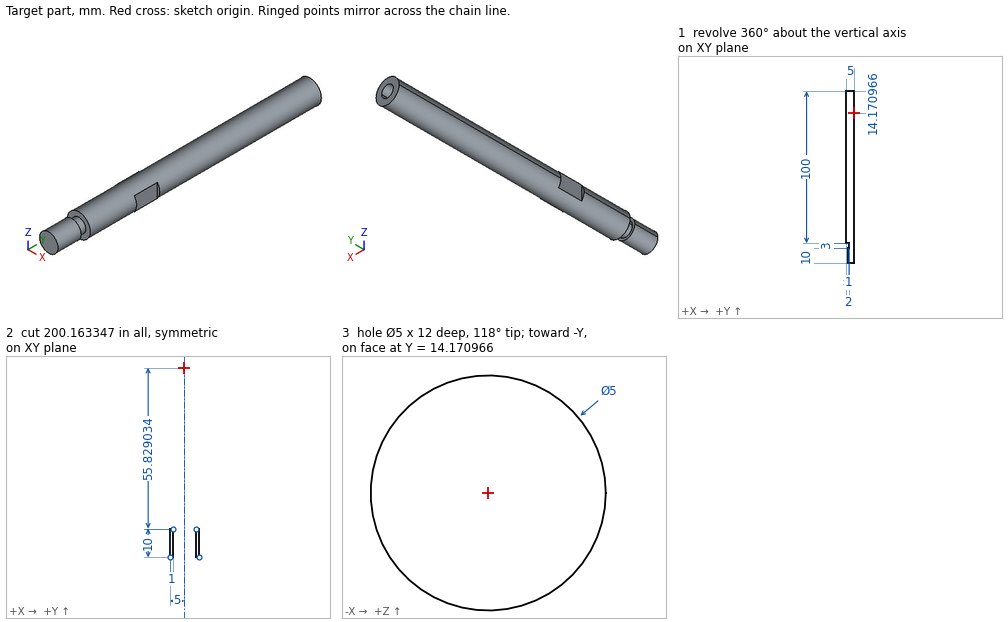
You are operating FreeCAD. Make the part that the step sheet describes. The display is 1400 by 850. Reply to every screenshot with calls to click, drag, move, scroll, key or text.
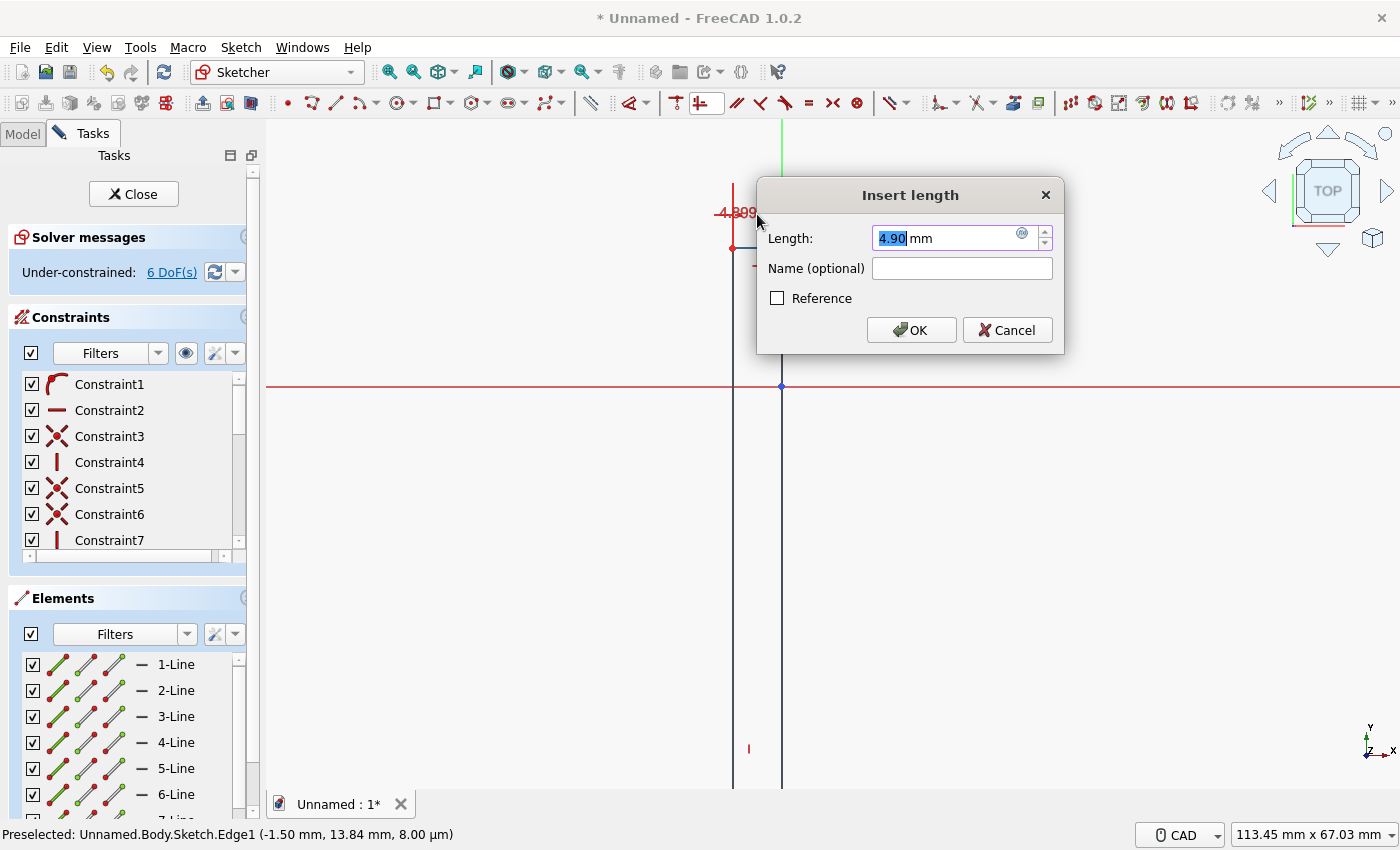
text(5)
key(Return)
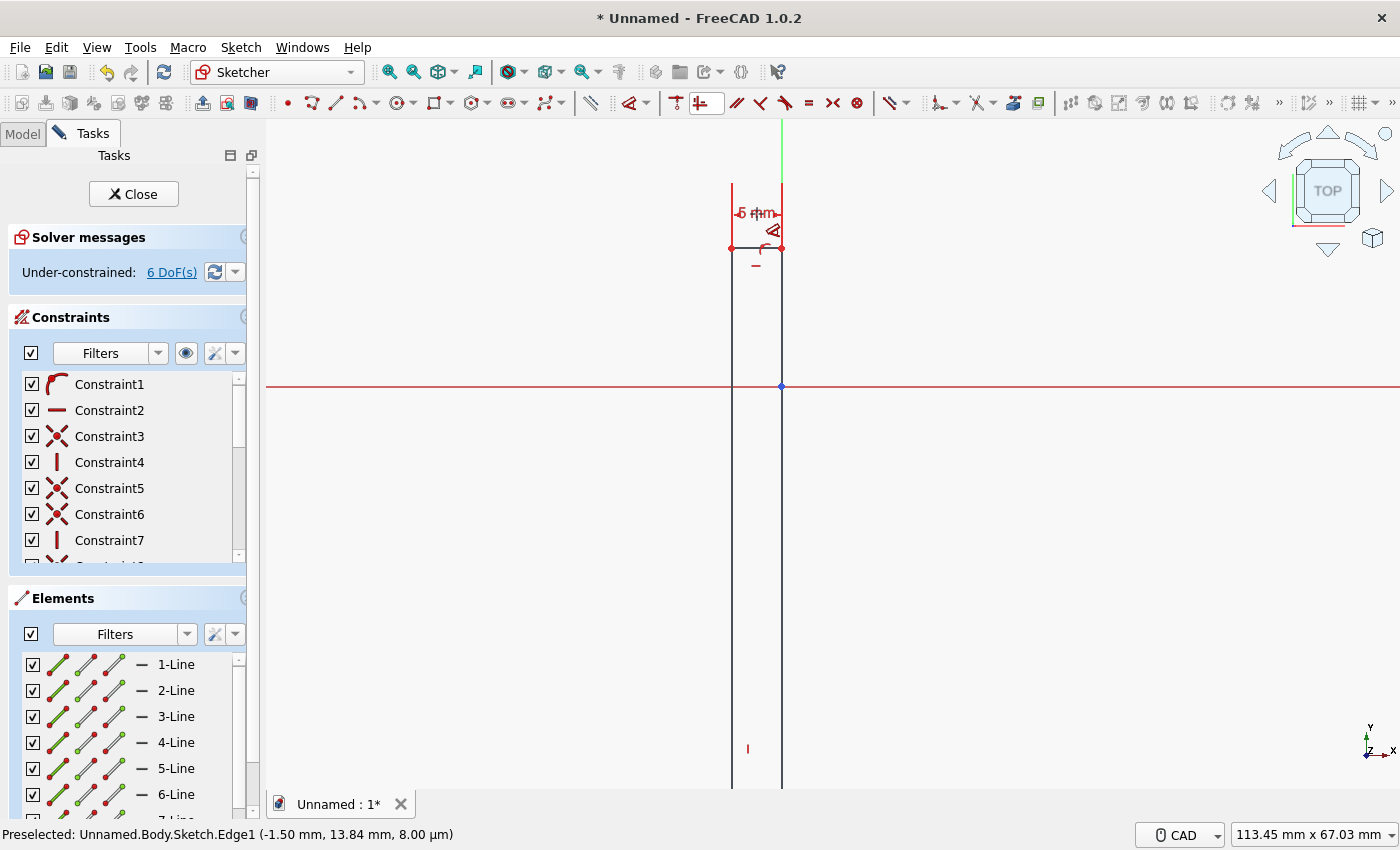
scroll(769, 247, down, 5)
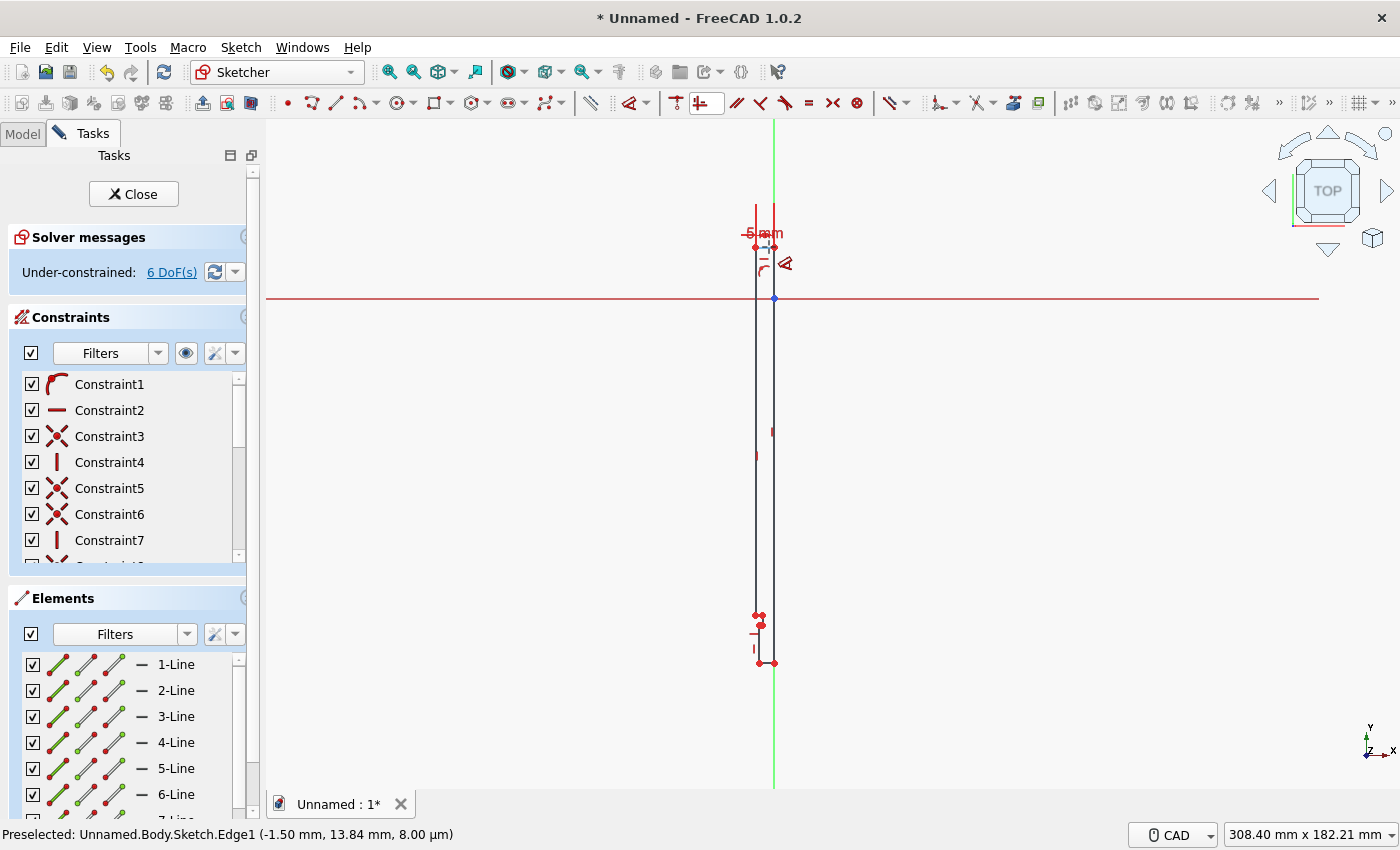
scroll(759, 616, up, 9)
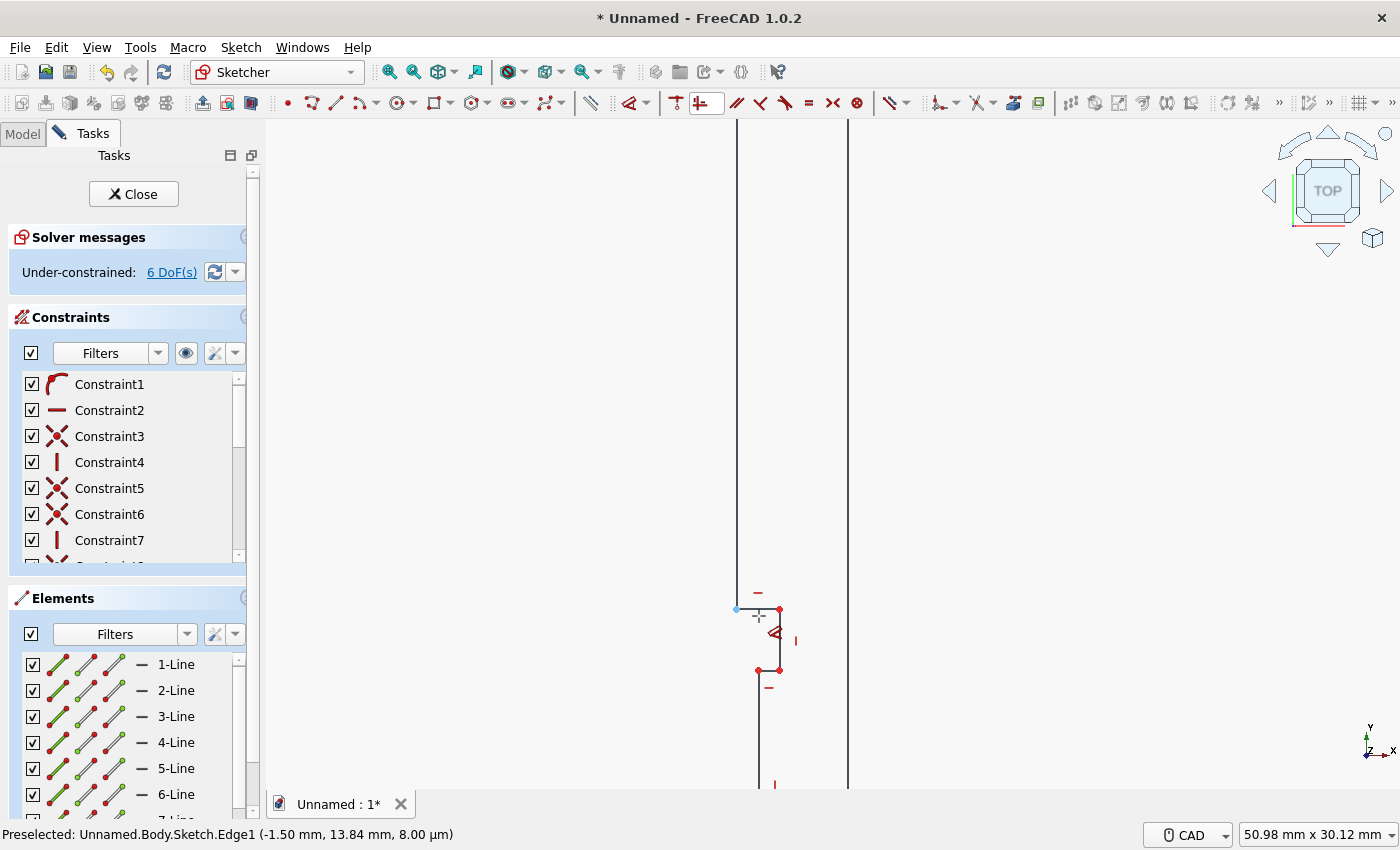
click(758, 609)
click(758, 643)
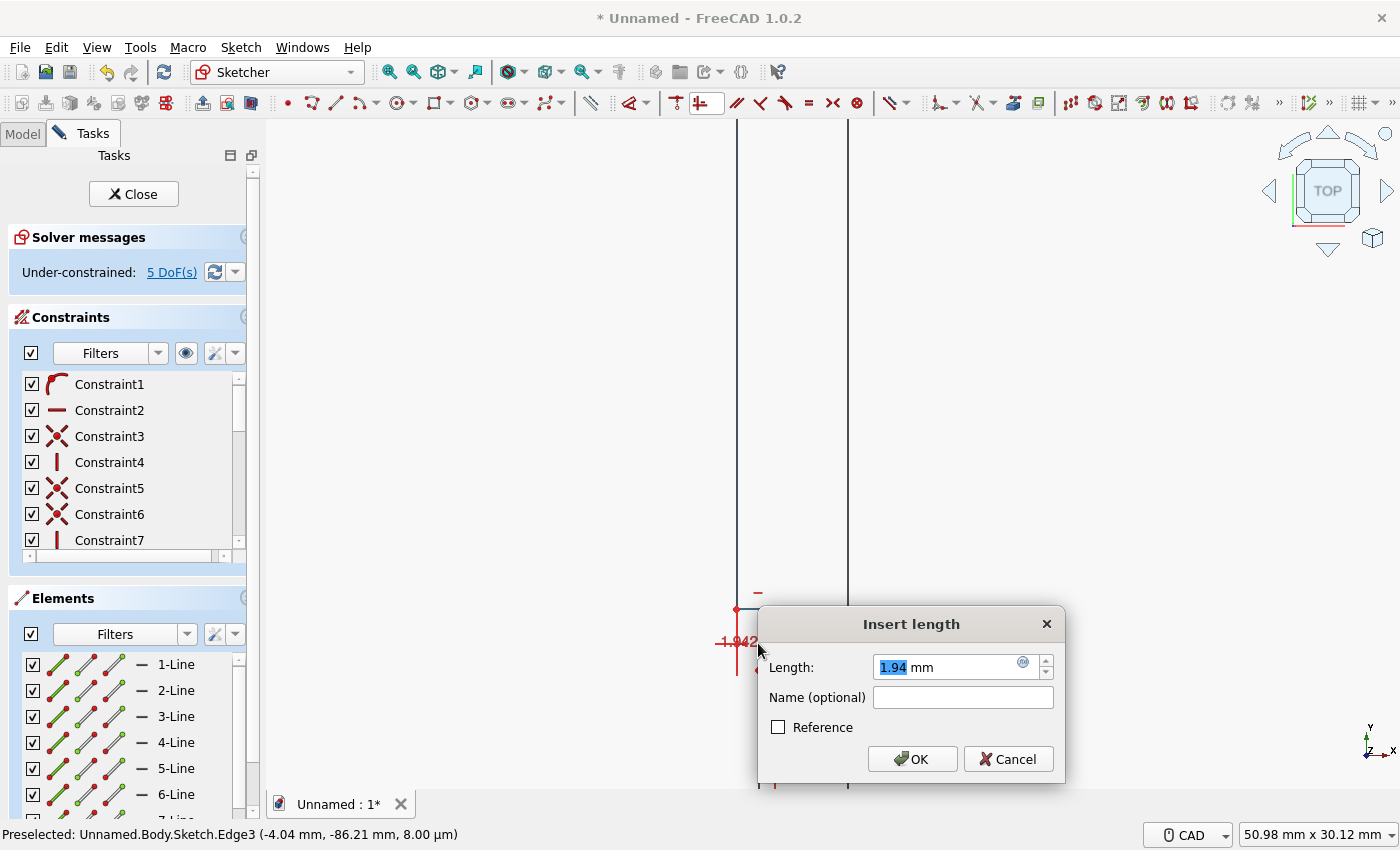
text(2)
key(Return)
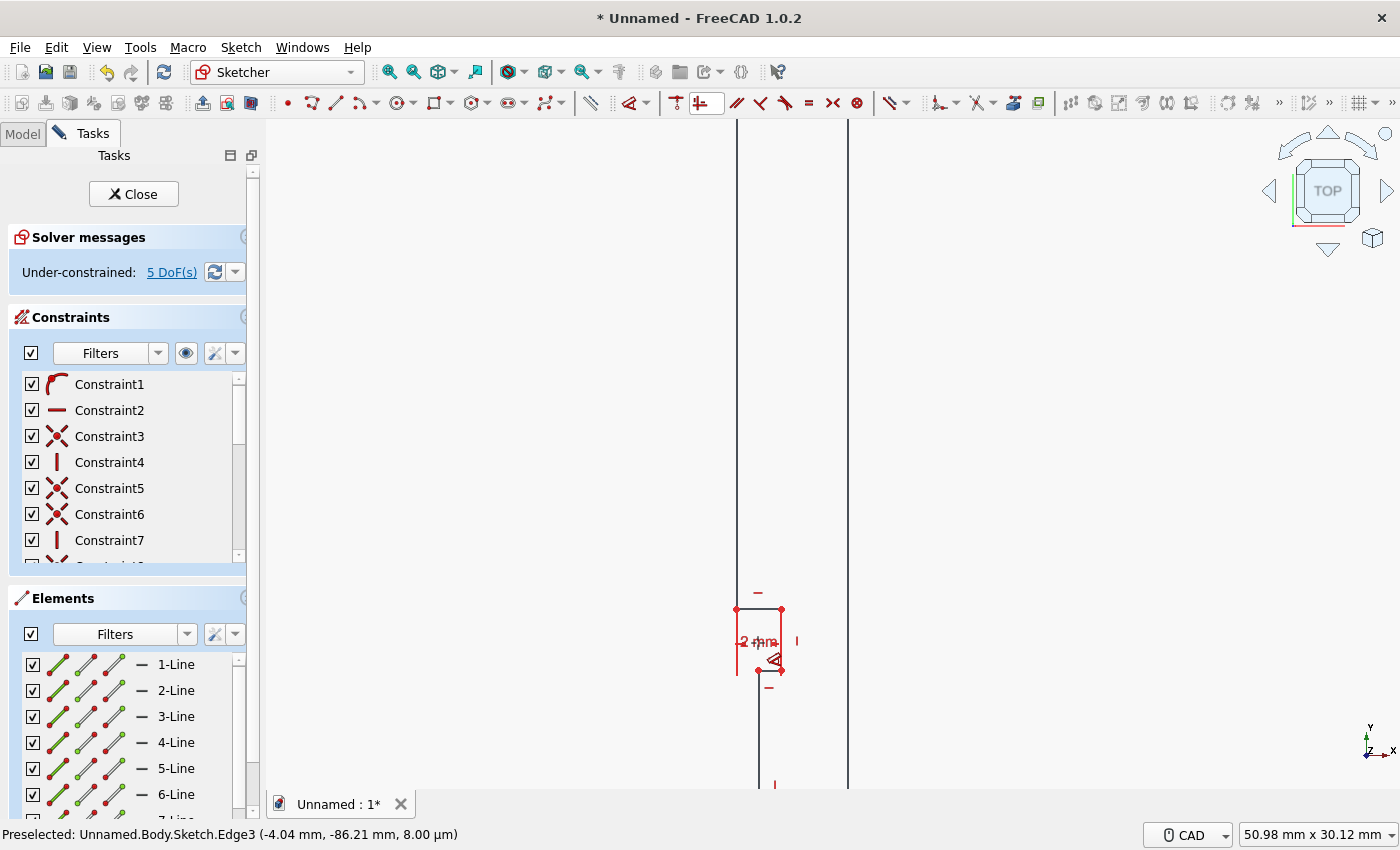
click(781, 628)
click(815, 619)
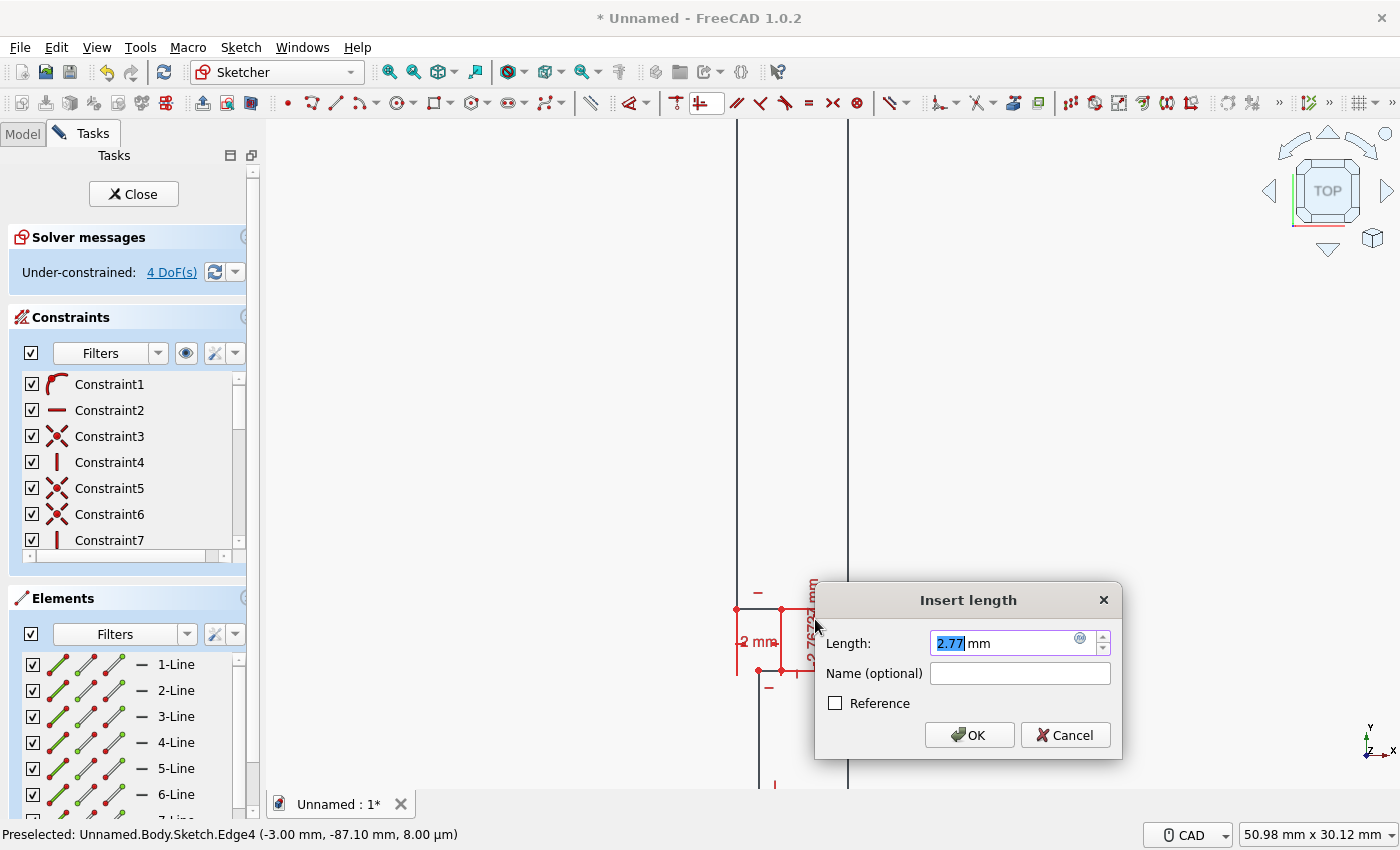
text(3)
key(Return)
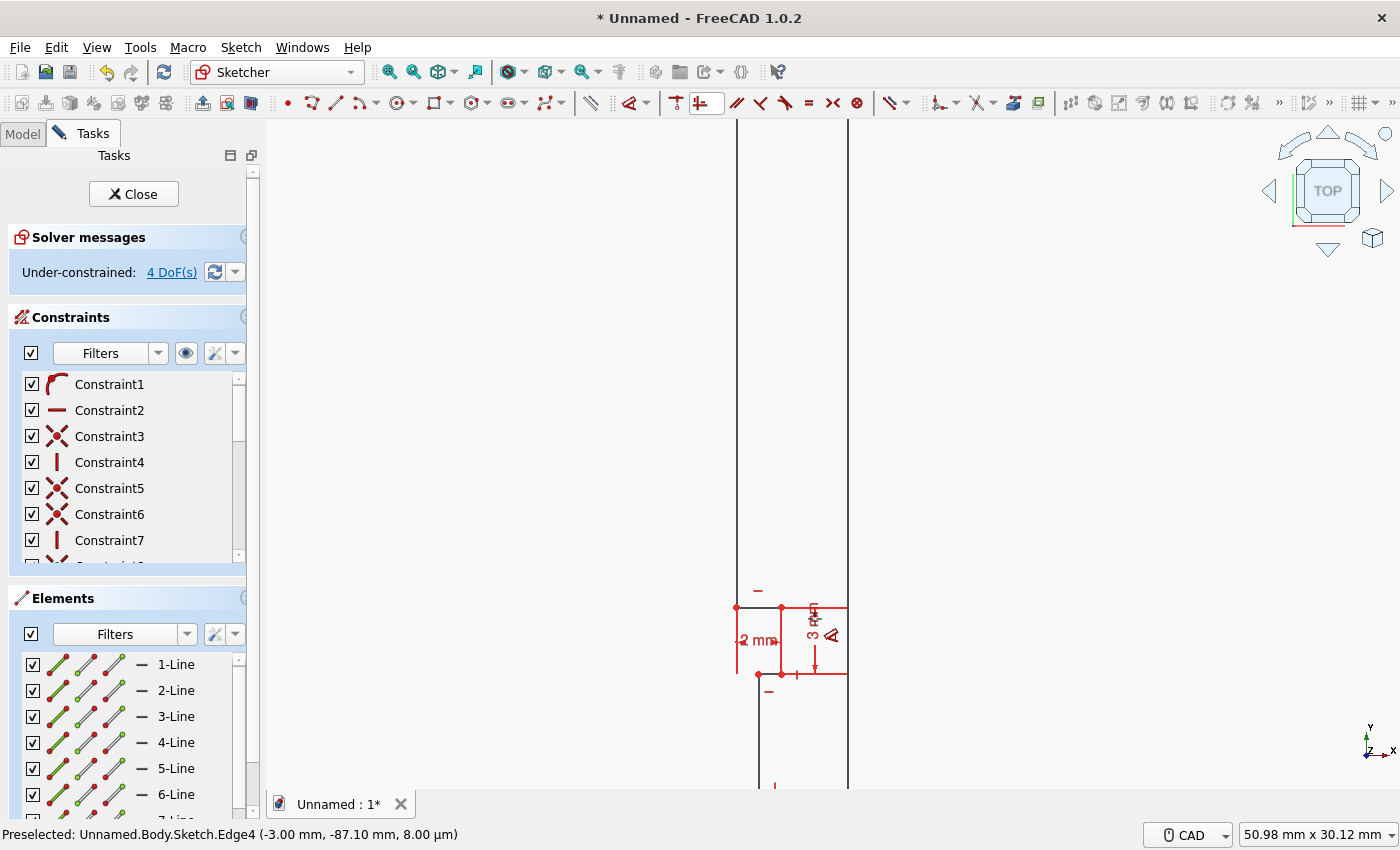
scroll(770, 674, up, 3)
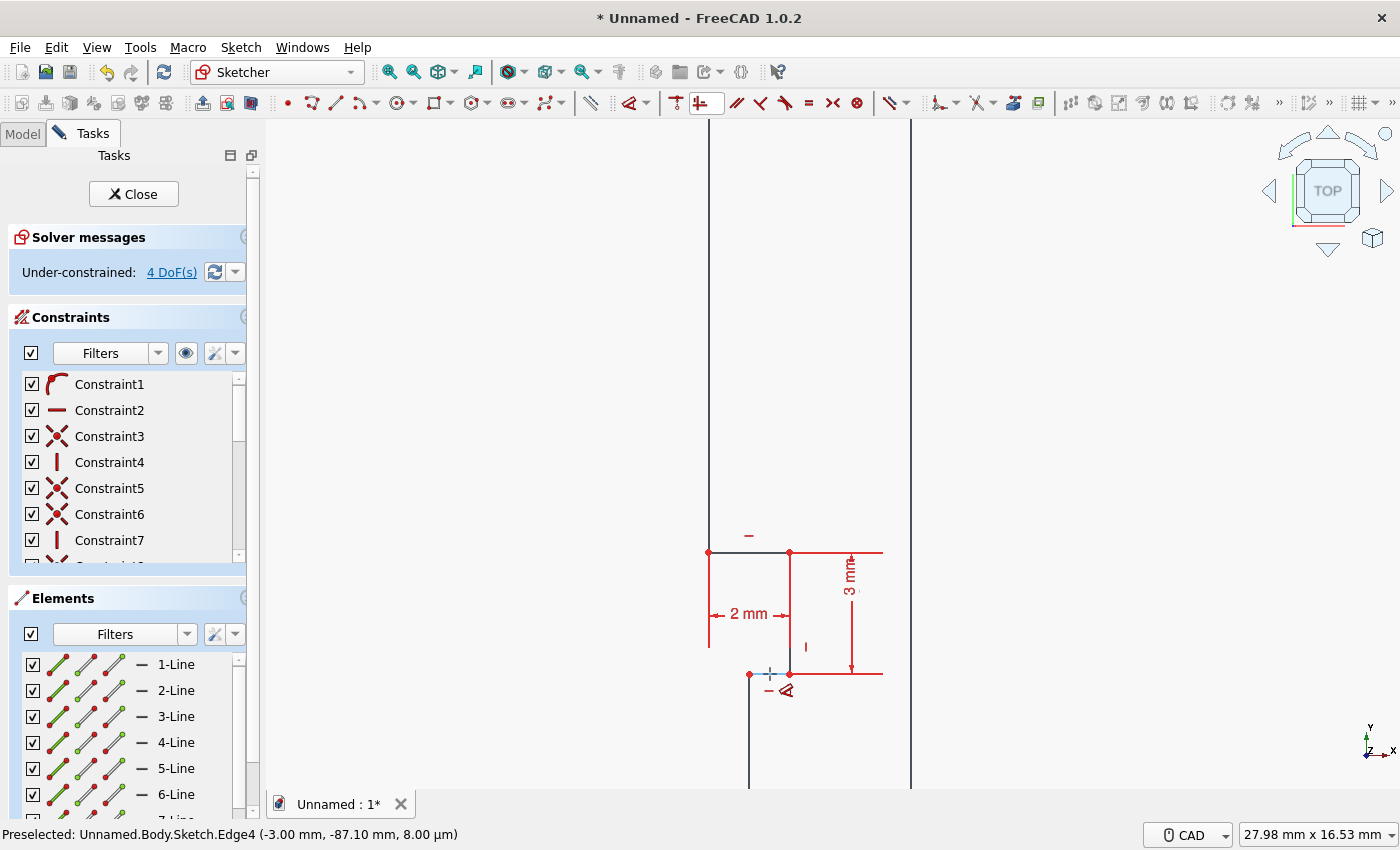
click(769, 674)
click(769, 708)